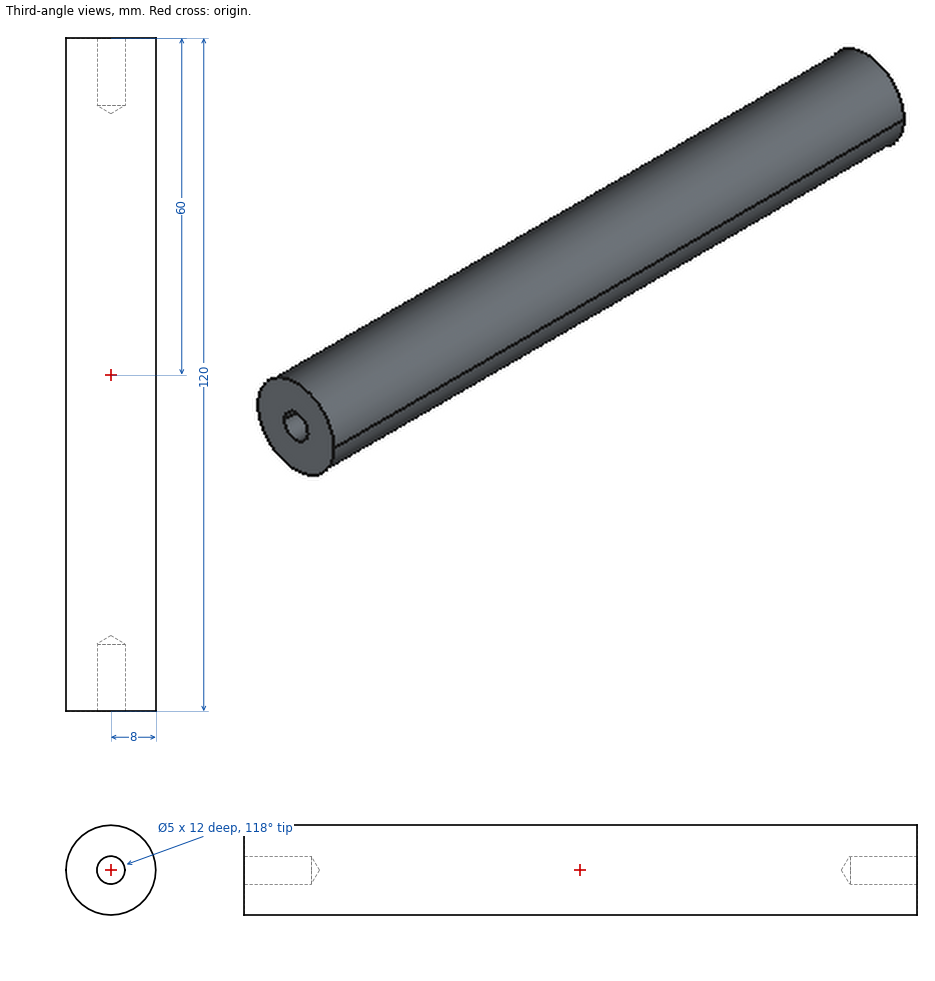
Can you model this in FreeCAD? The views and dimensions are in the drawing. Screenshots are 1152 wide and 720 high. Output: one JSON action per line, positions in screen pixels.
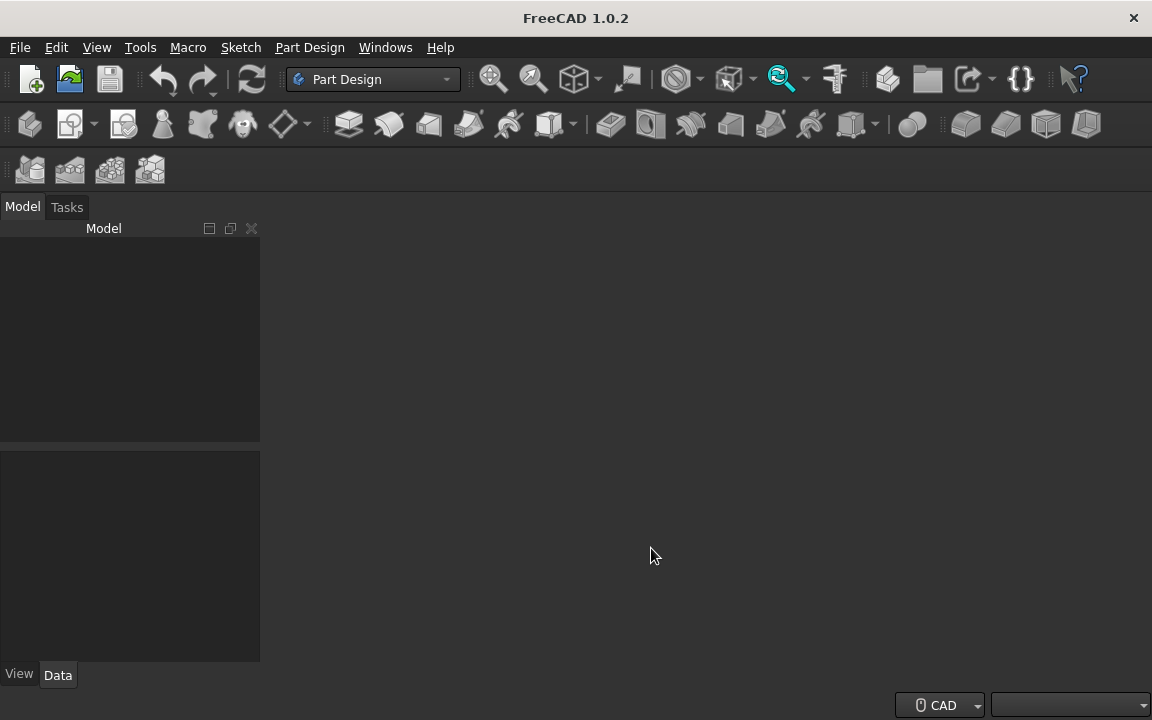
{"action": "key", "text": "ctrl+n"}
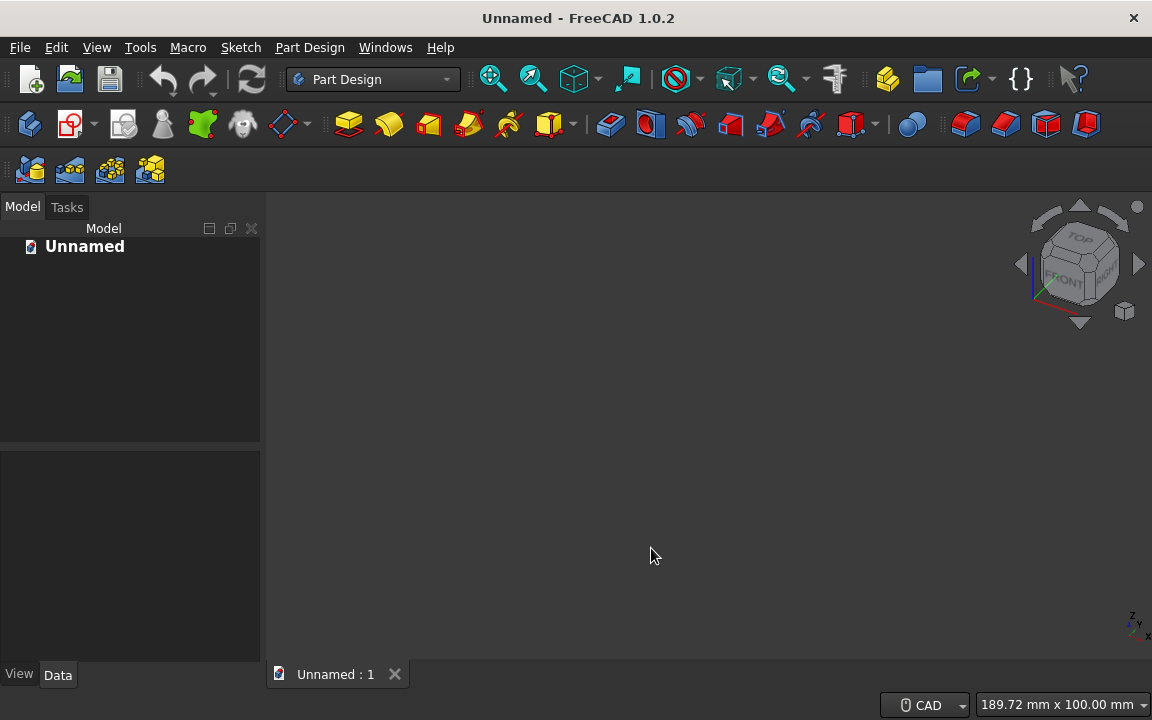
{"action": "left_click", "coordinate": [70, 124]}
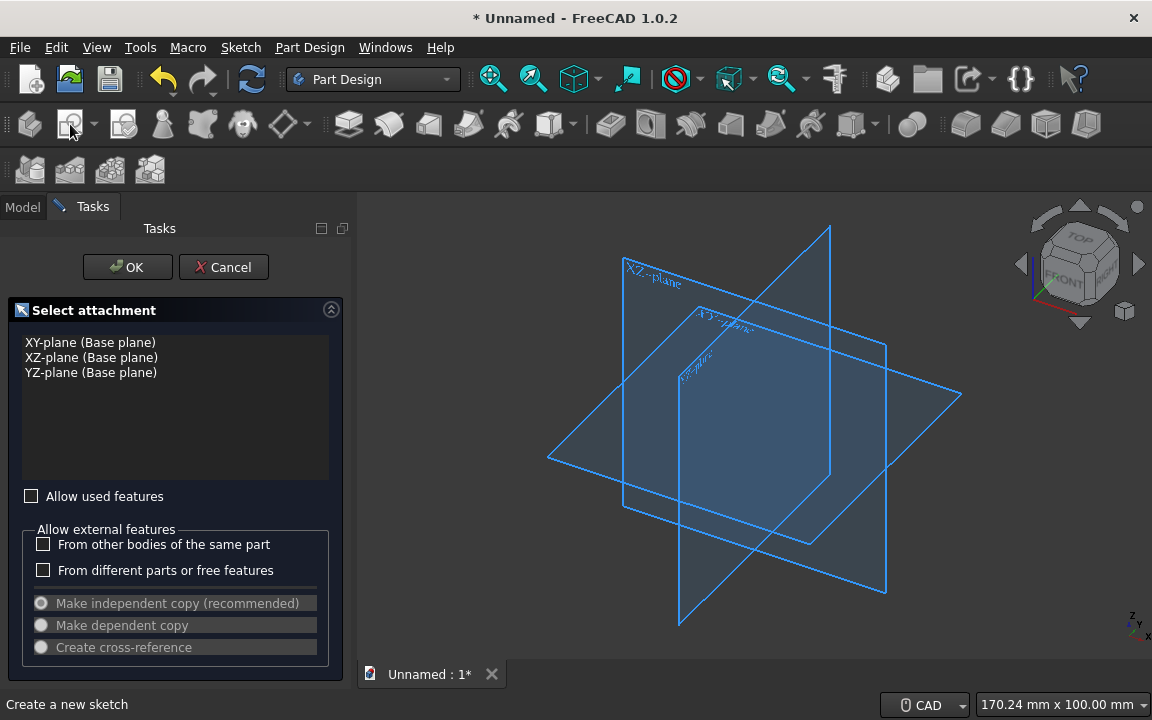
{"action": "left_click", "coordinate": [82, 342]}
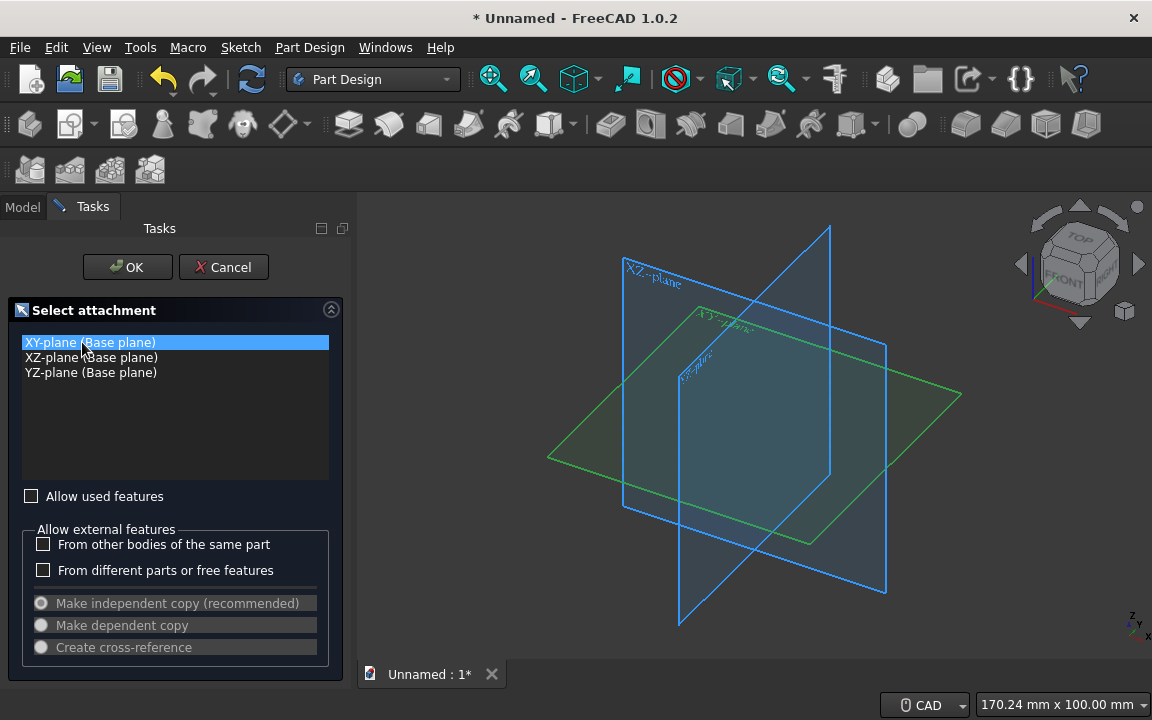
{"action": "left_click", "coordinate": [128, 267]}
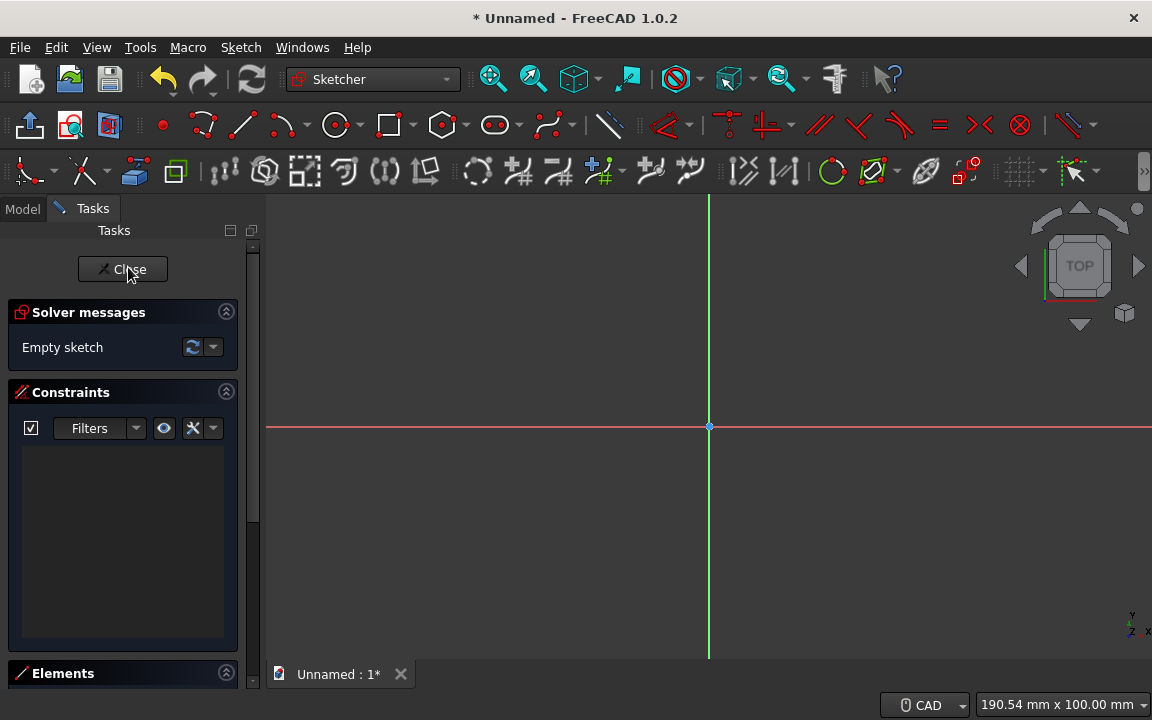
{"action": "scroll", "coordinate": [535, 426], "scroll_direction": "down", "scroll_amount": 3}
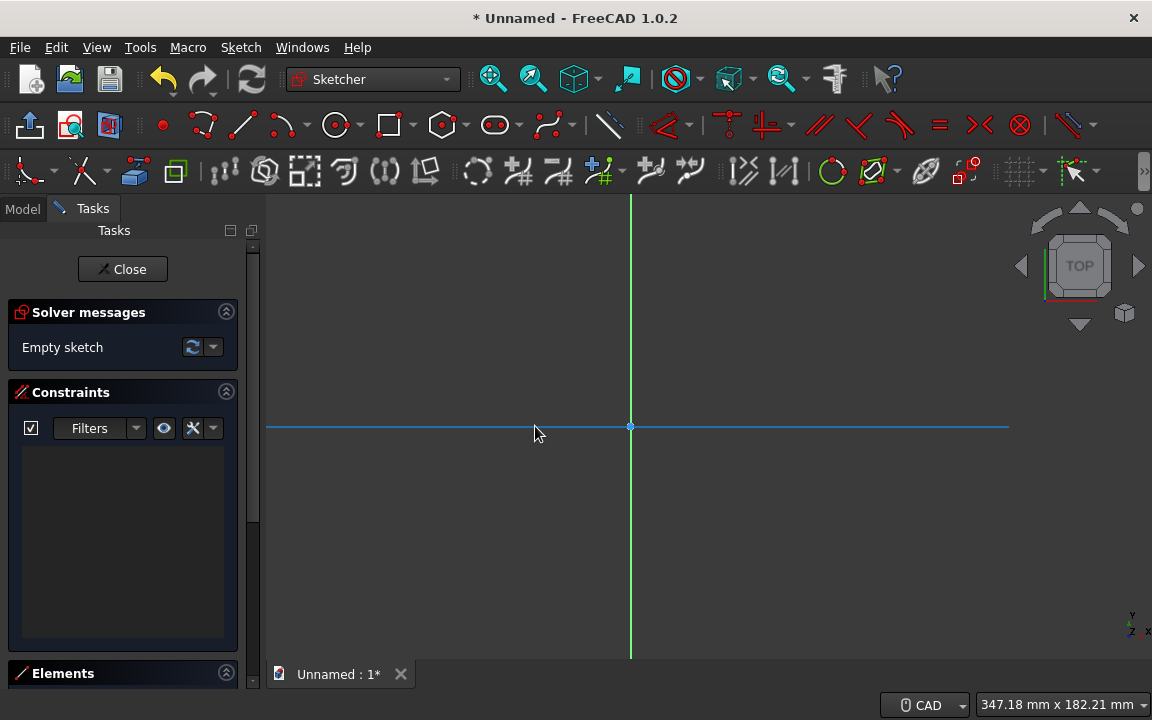
{"action": "key", "text": "g r"}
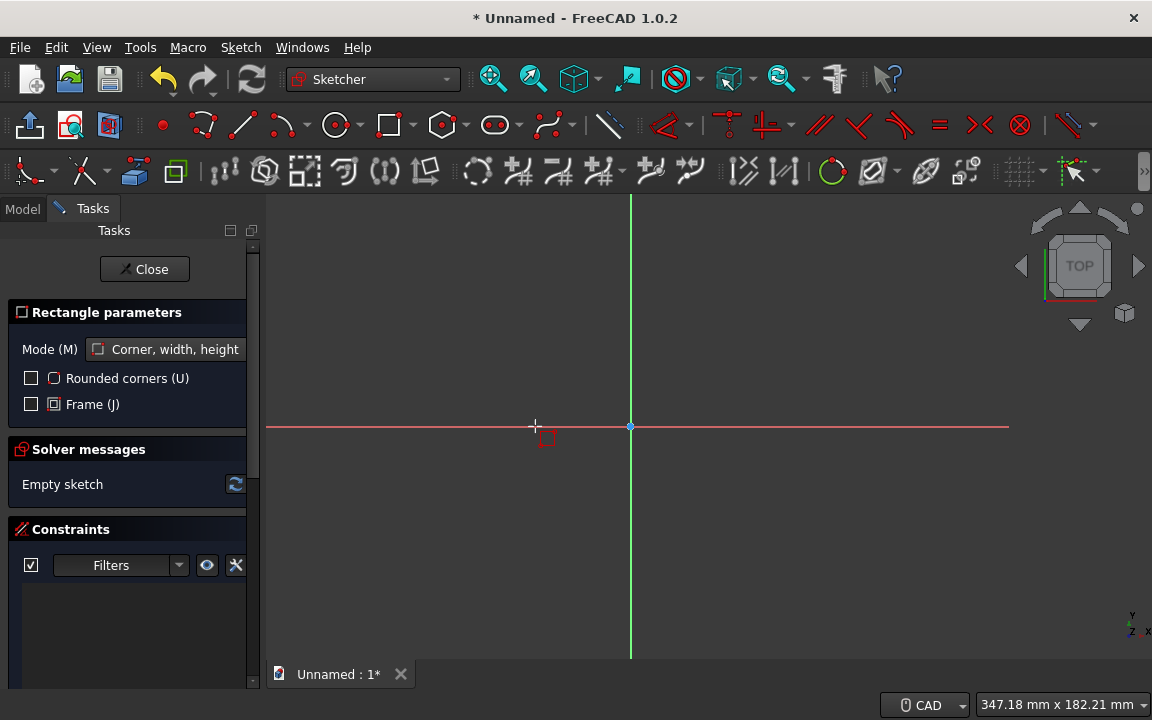
{"action": "left_click", "coordinate": [631, 273]}
{"action": "left_click", "coordinate": [651, 580]}
{"action": "key", "text": "Escape"}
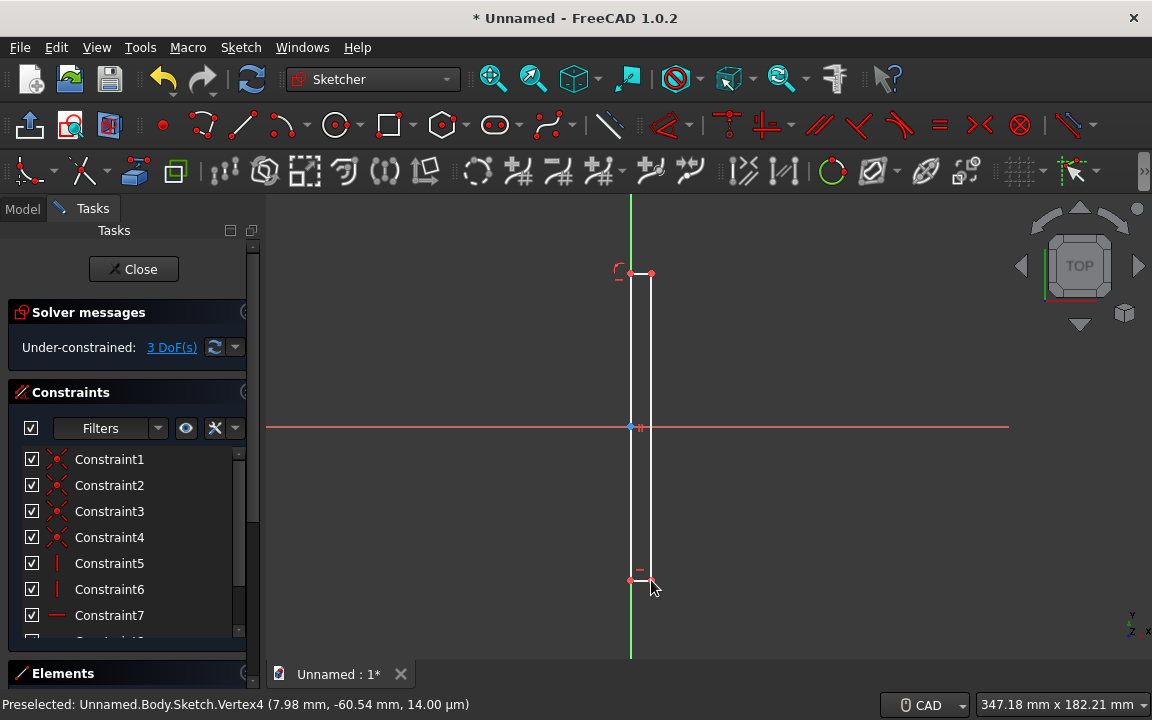
{"action": "scroll", "coordinate": [641, 581], "scroll_direction": "up", "scroll_amount": 4}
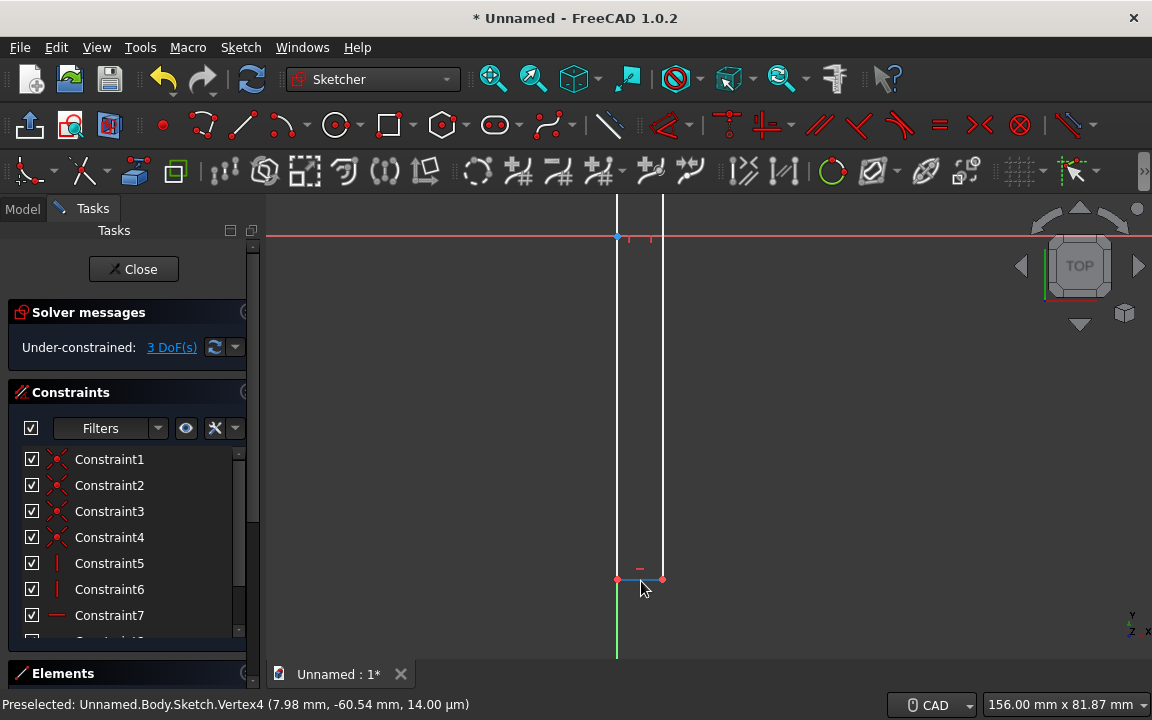
{"action": "left_click", "coordinate": [640, 580]}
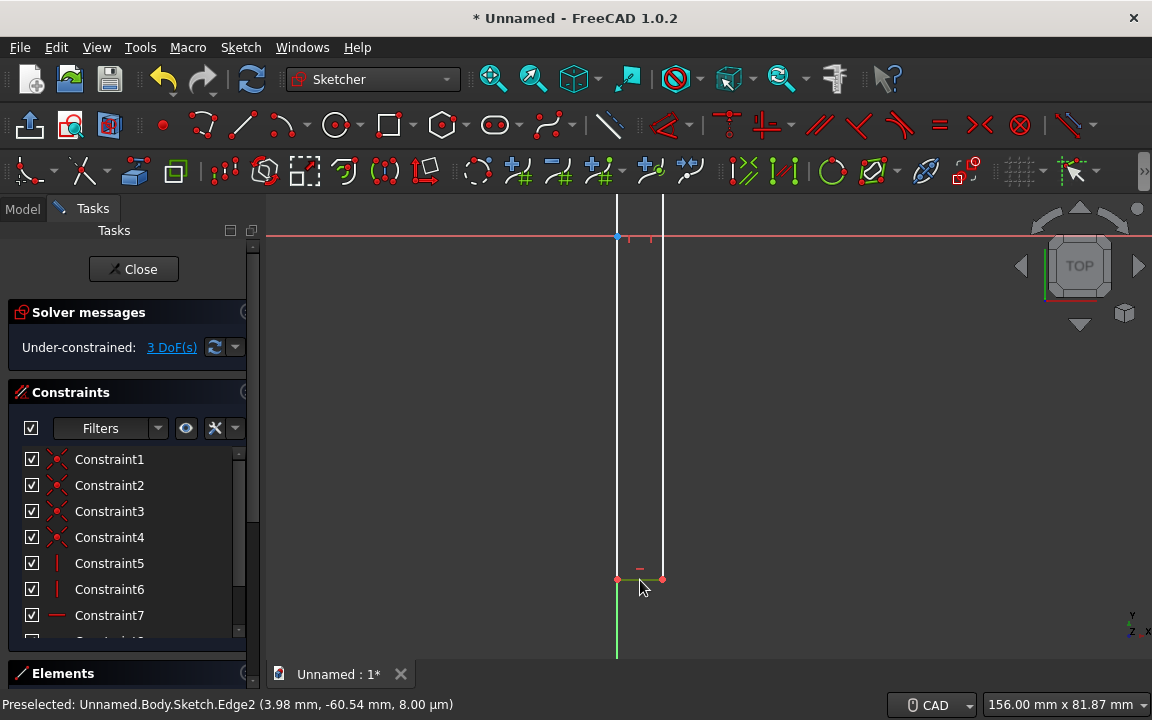
{"action": "key", "text": "l"}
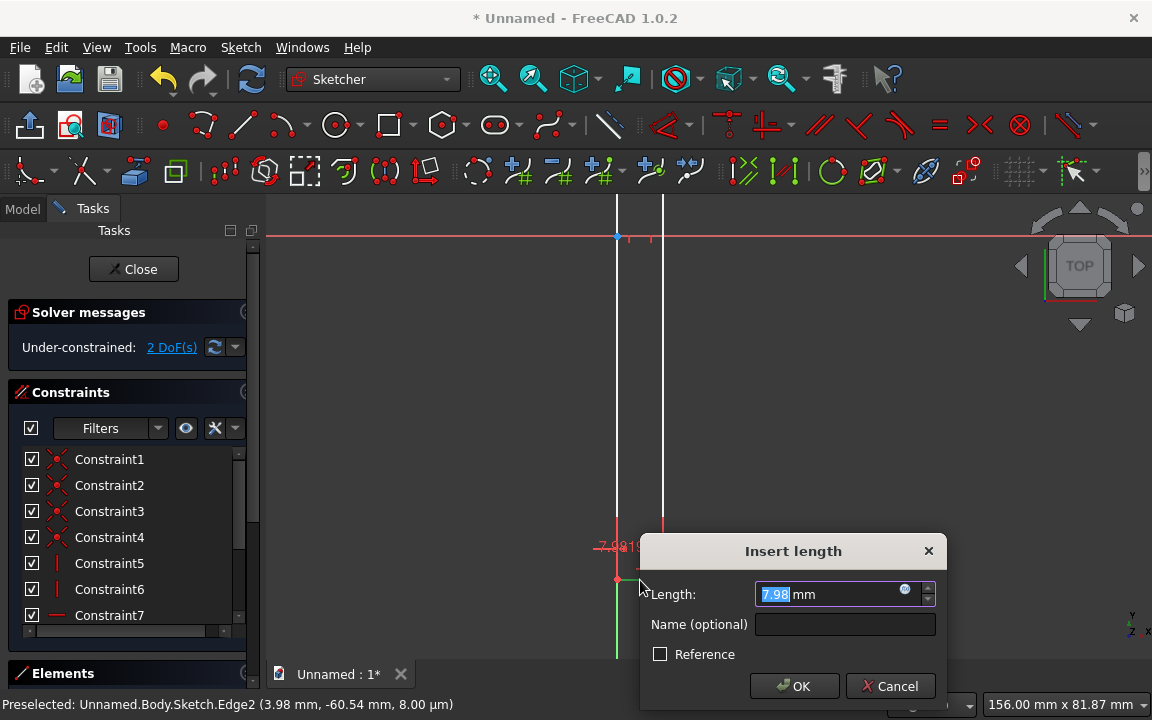
{"action": "type", "text": "8"}
{"action": "key", "text": "Return"}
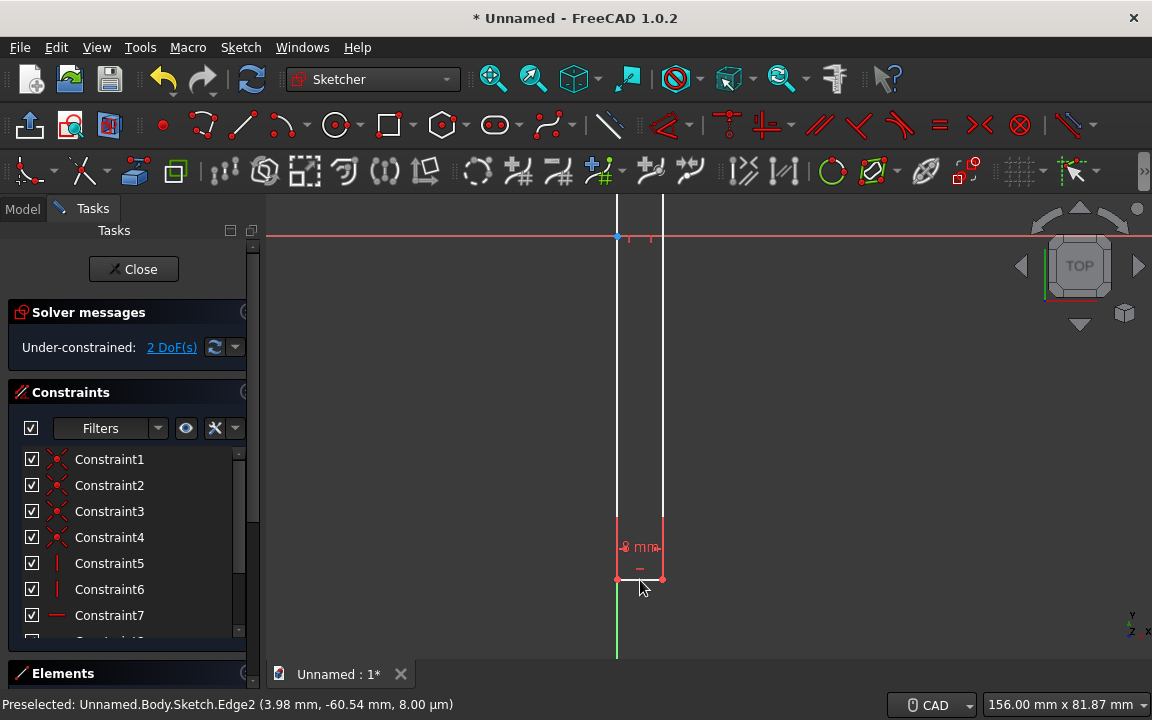
{"action": "left_click", "coordinate": [617, 375]}